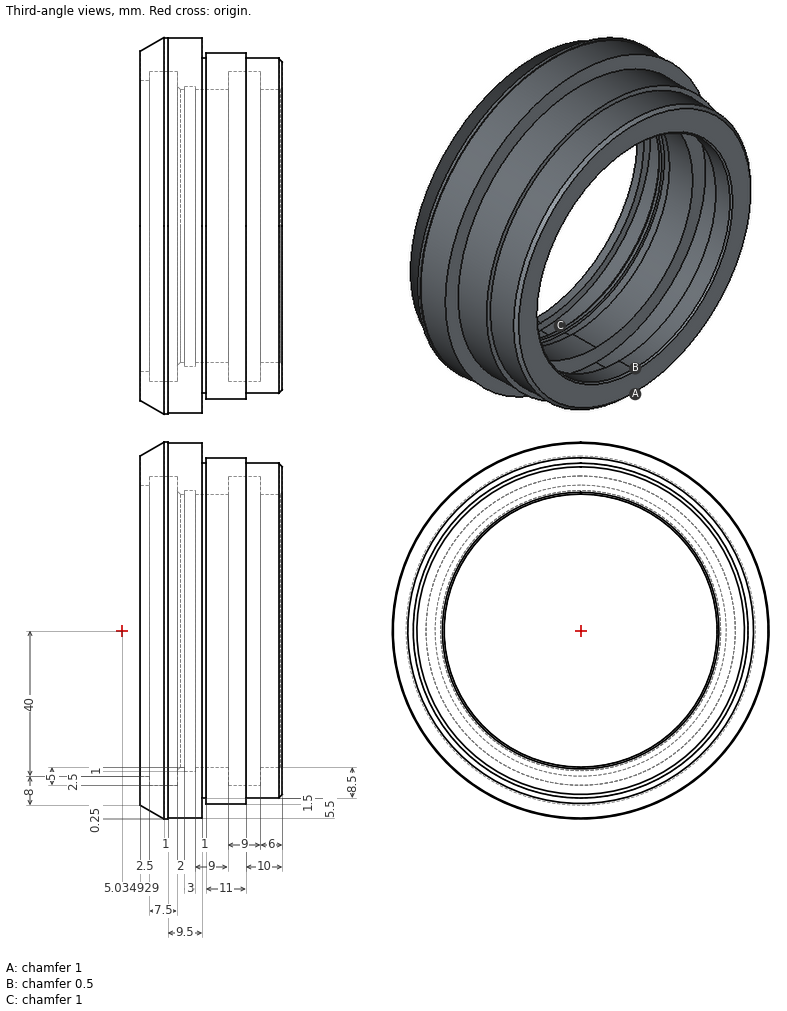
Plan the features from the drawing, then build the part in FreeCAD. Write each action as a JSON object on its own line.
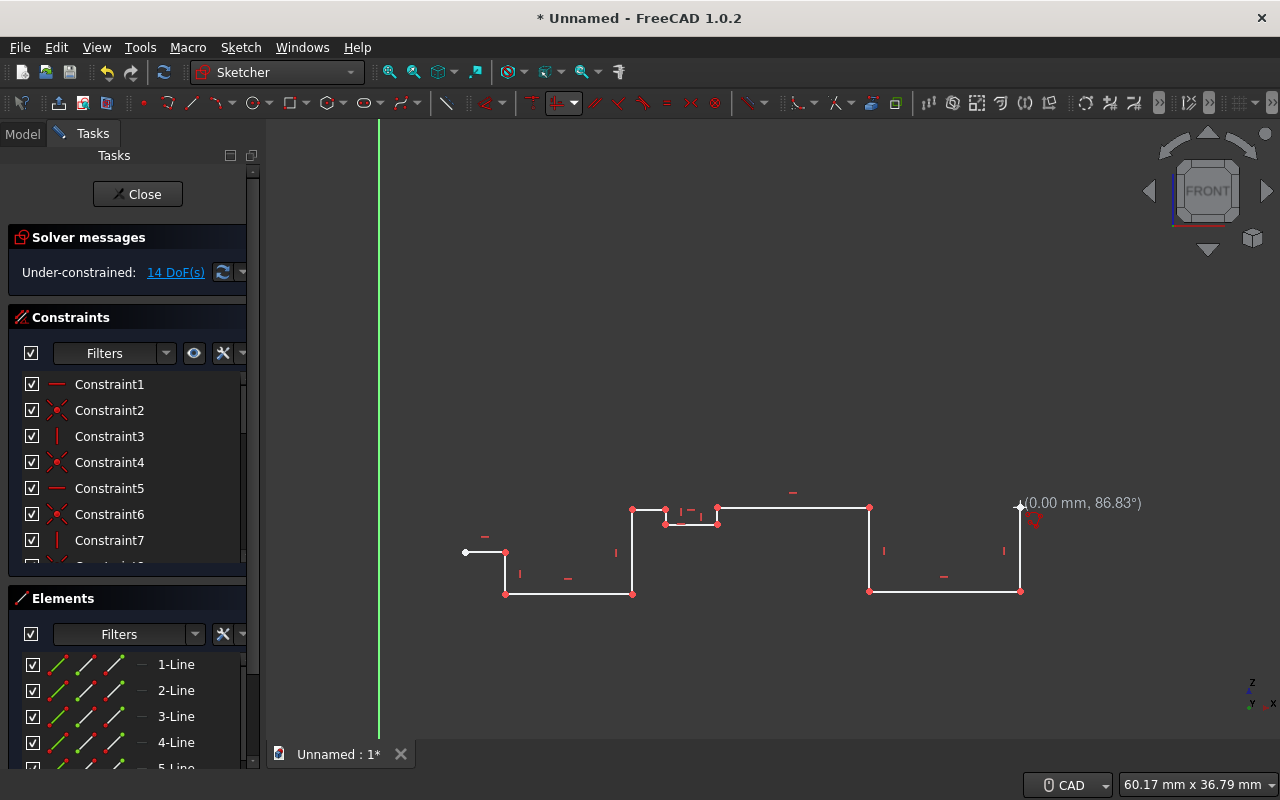
{"action": "scroll", "coordinate": [667, 525], "scroll_direction": "down", "scroll_amount": 4}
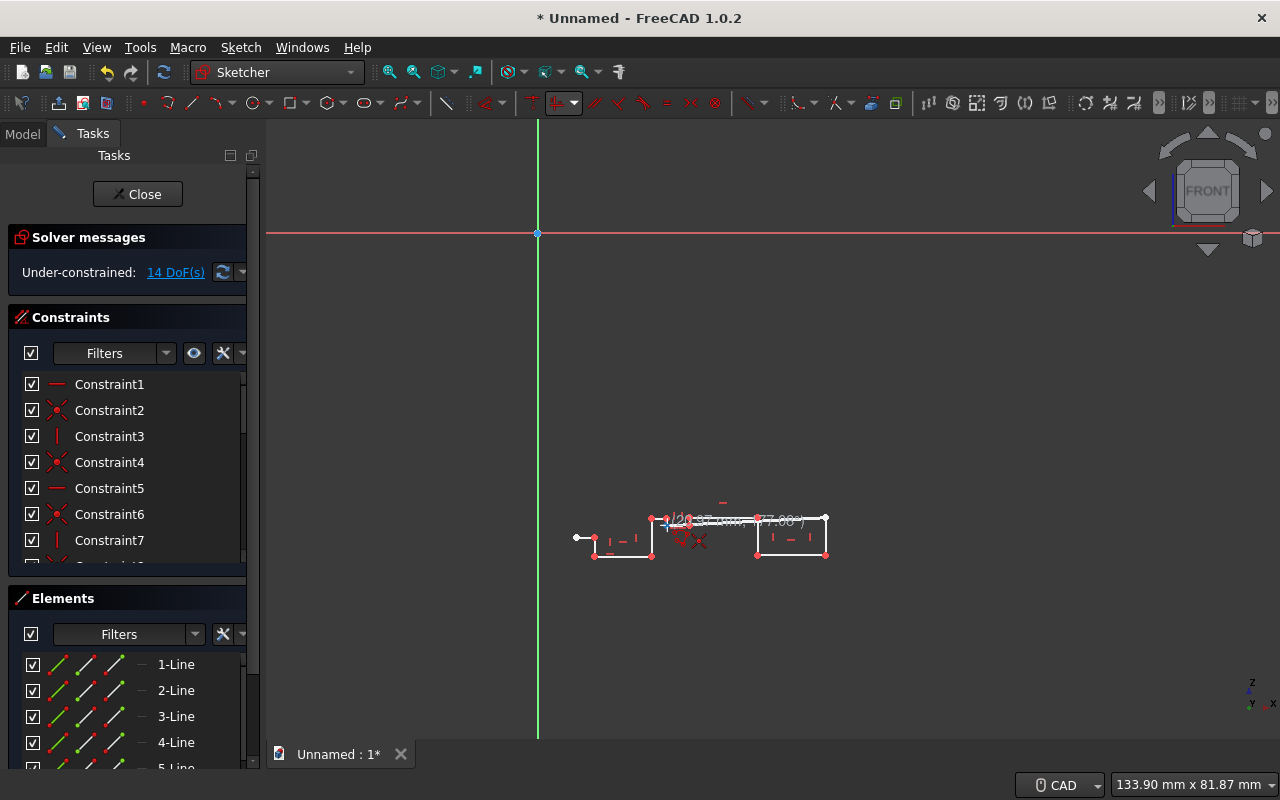
{"action": "left_click", "coordinate": [871, 517]}
{"action": "left_click", "coordinate": [871, 582]}
{"action": "left_click", "coordinate": [796, 582]}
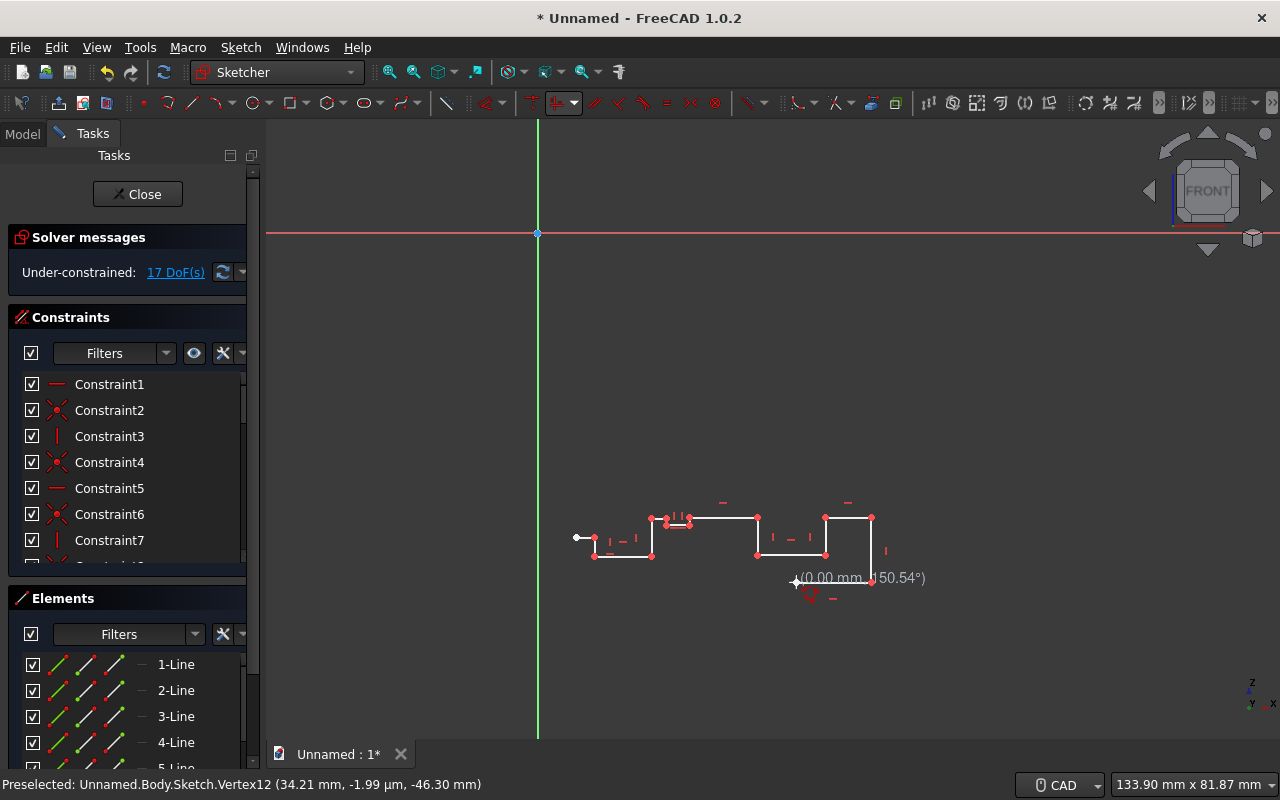
{"action": "scroll", "coordinate": [796, 593], "scroll_direction": "up", "scroll_amount": 2}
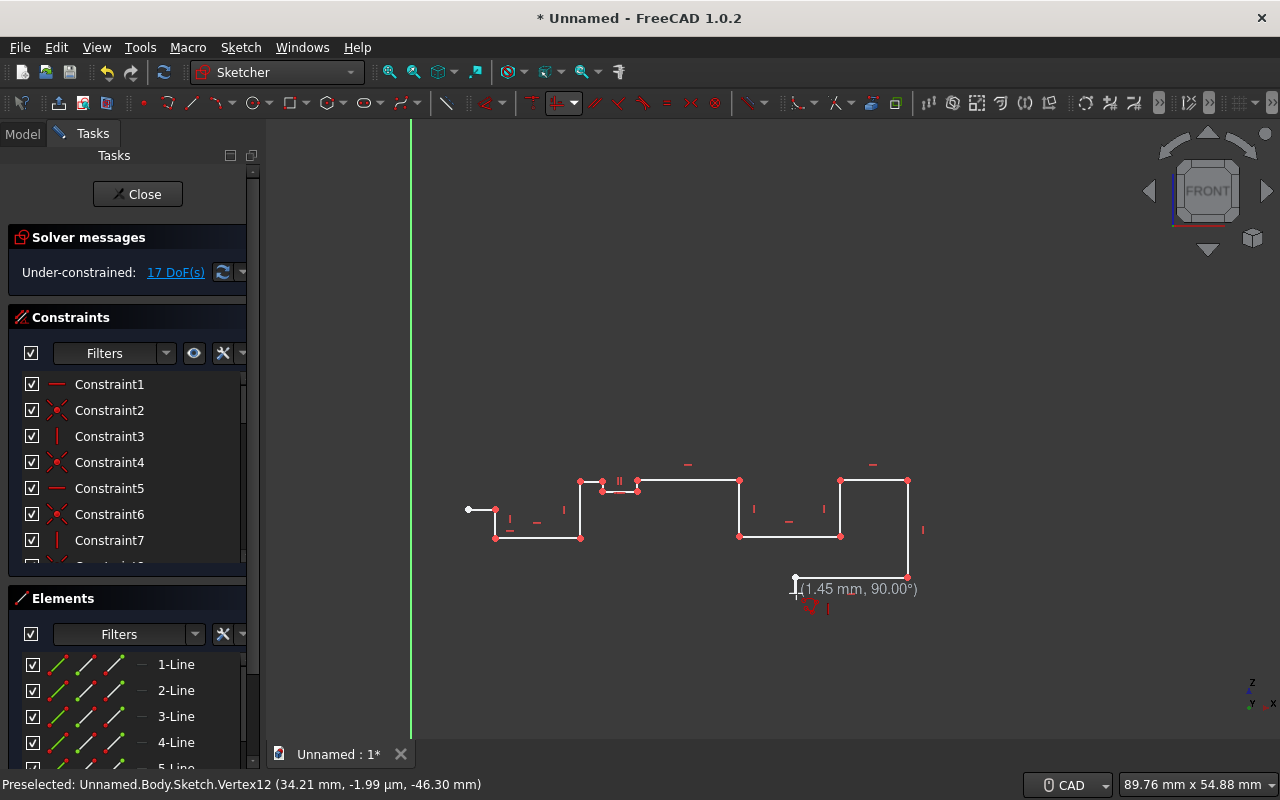
{"action": "left_click", "coordinate": [796, 593]}
{"action": "left_click", "coordinate": [671, 593]}
{"action": "left_click", "coordinate": [671, 576]}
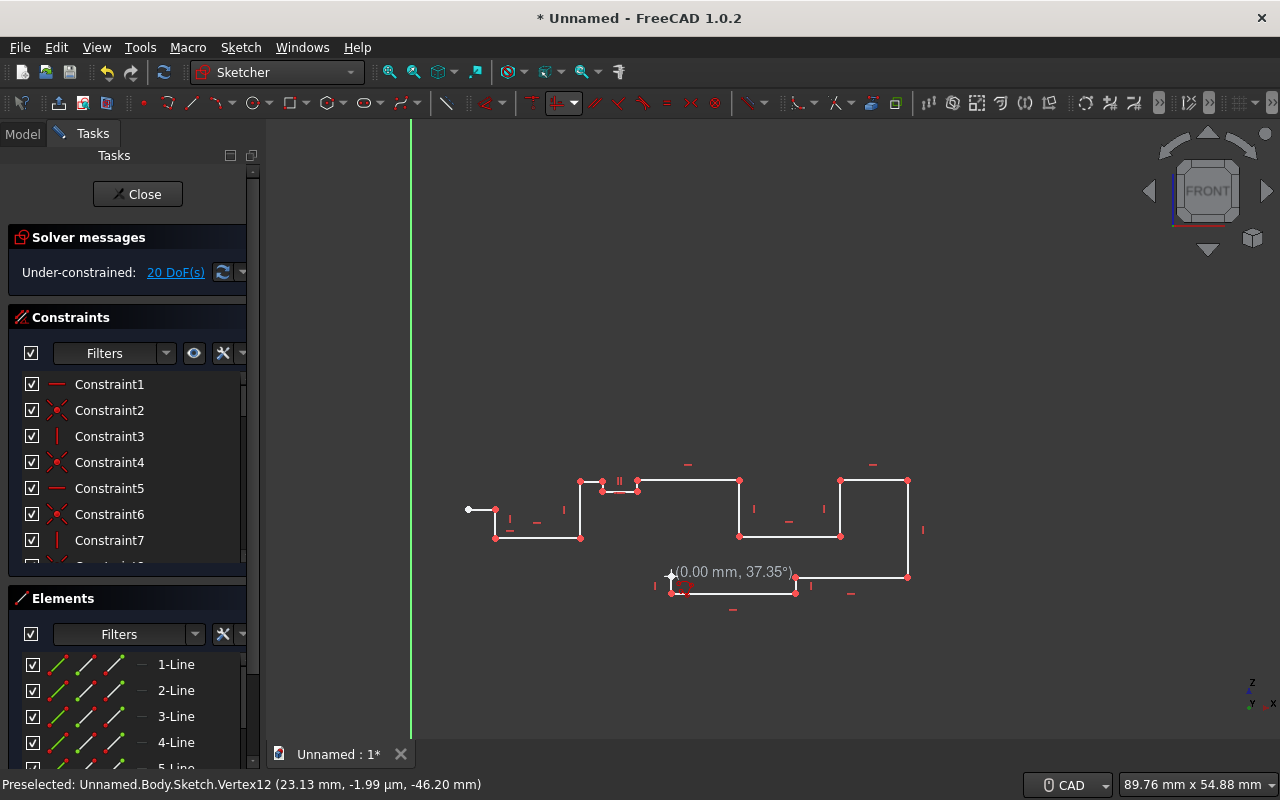
{"action": "scroll", "coordinate": [660, 576], "scroll_direction": "up", "scroll_amount": 2}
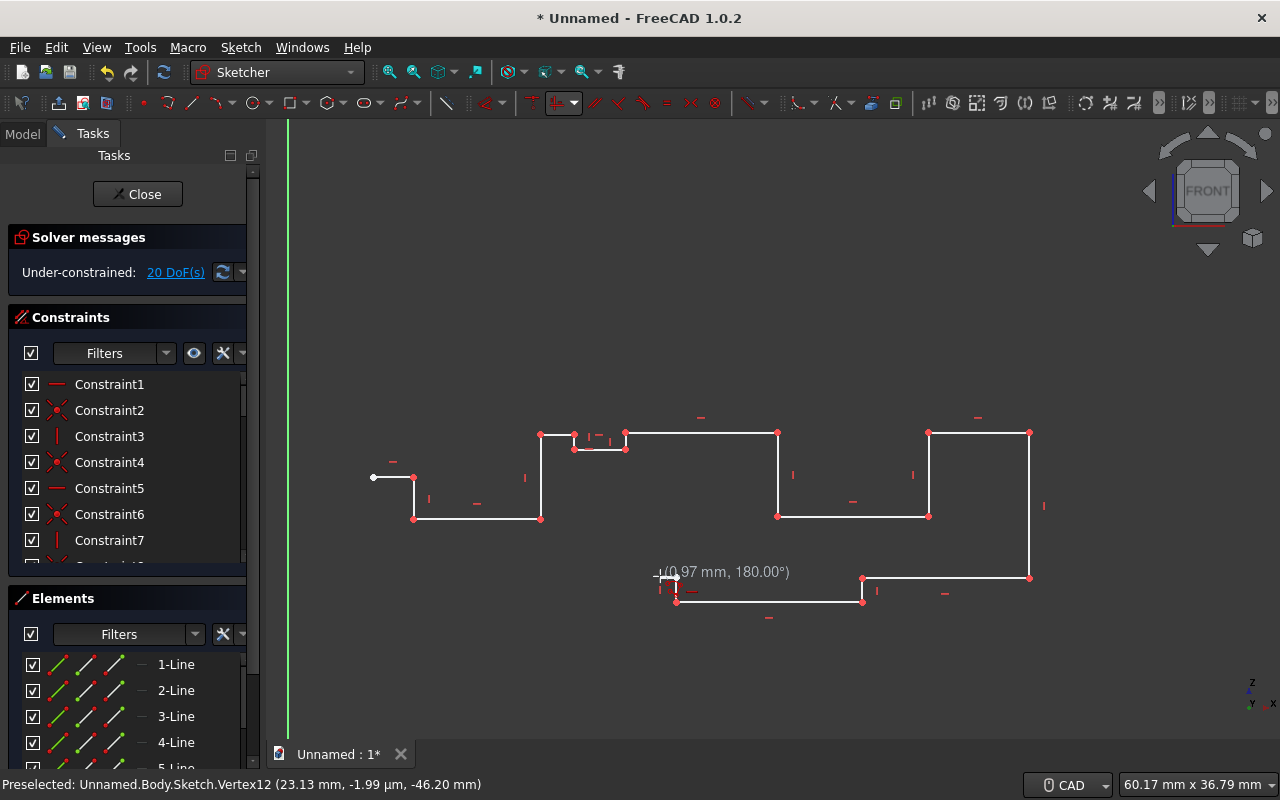
{"action": "left_click", "coordinate": [659, 576]}
{"action": "left_click", "coordinate": [659, 668]}
{"action": "left_click", "coordinate": [499, 668]}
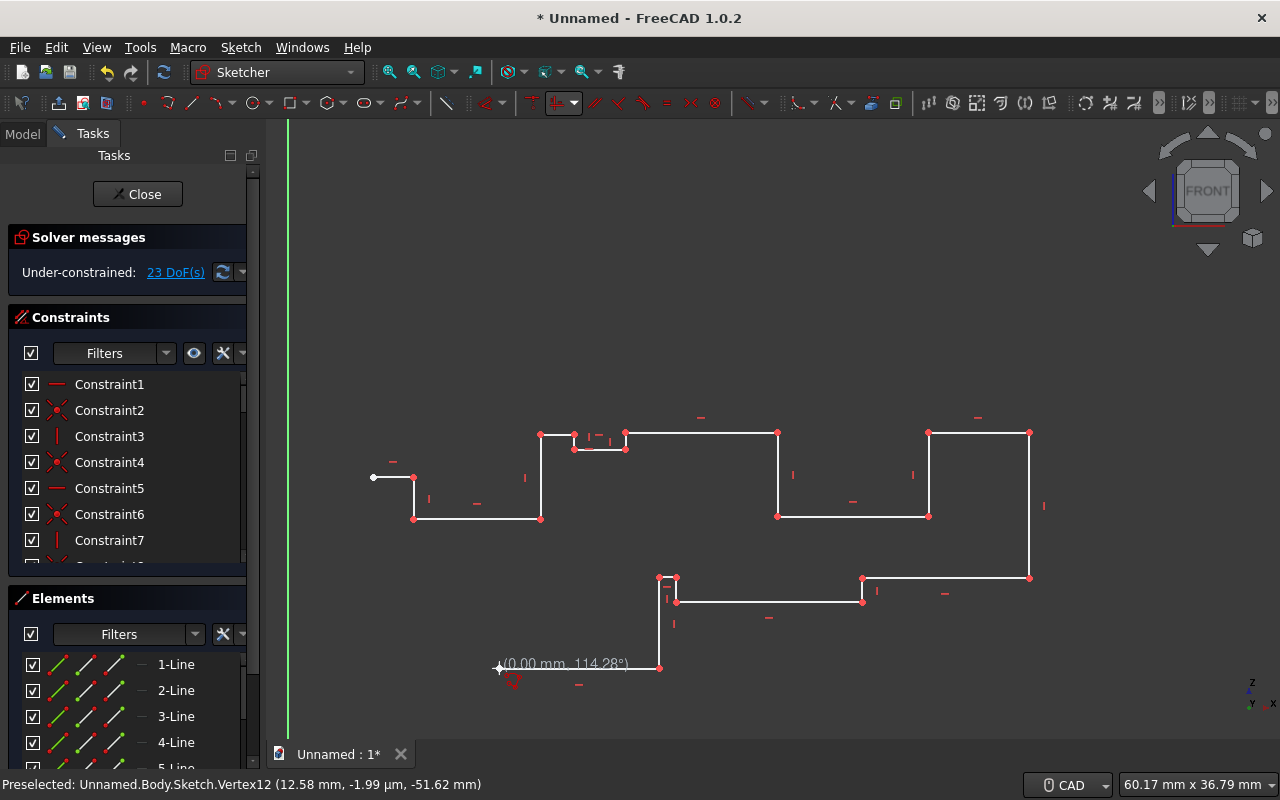
{"action": "scroll", "coordinate": [499, 672], "scroll_direction": "up", "scroll_amount": 7}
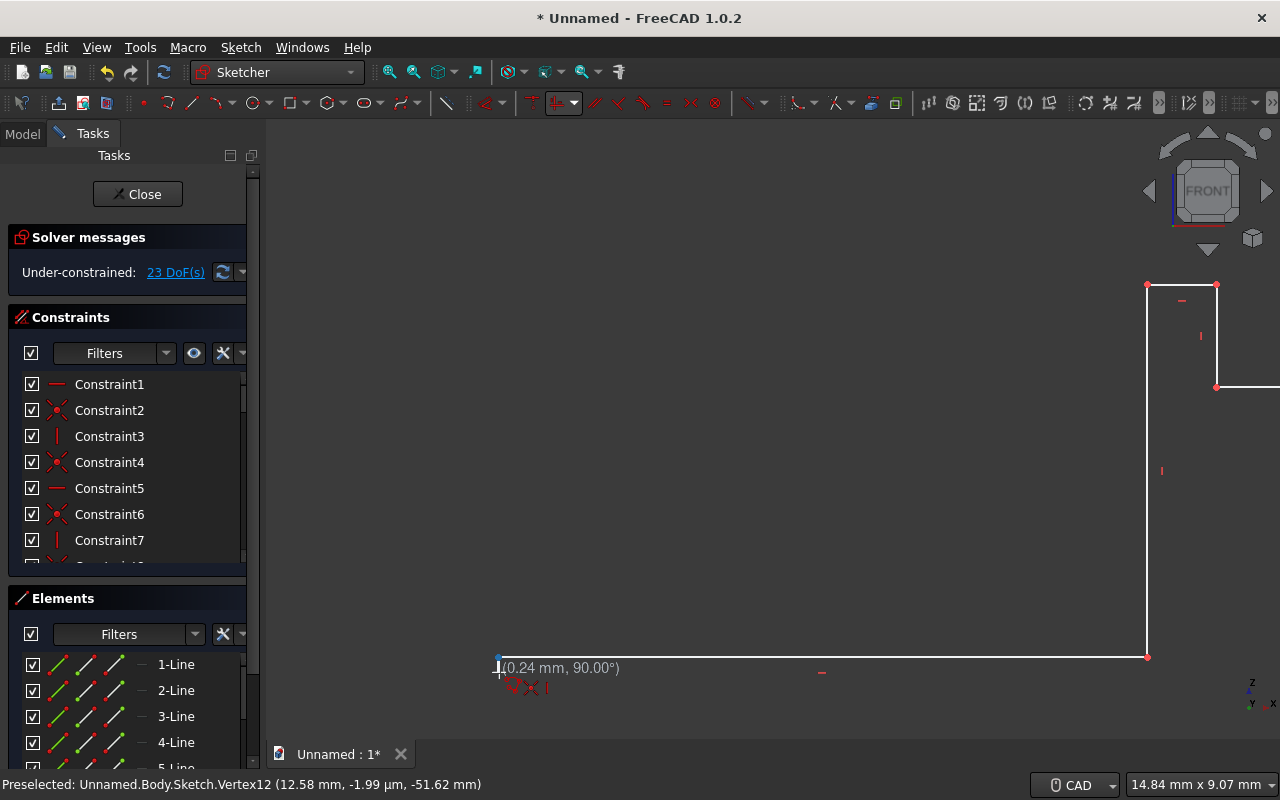
{"action": "left_click", "coordinate": [498, 670]}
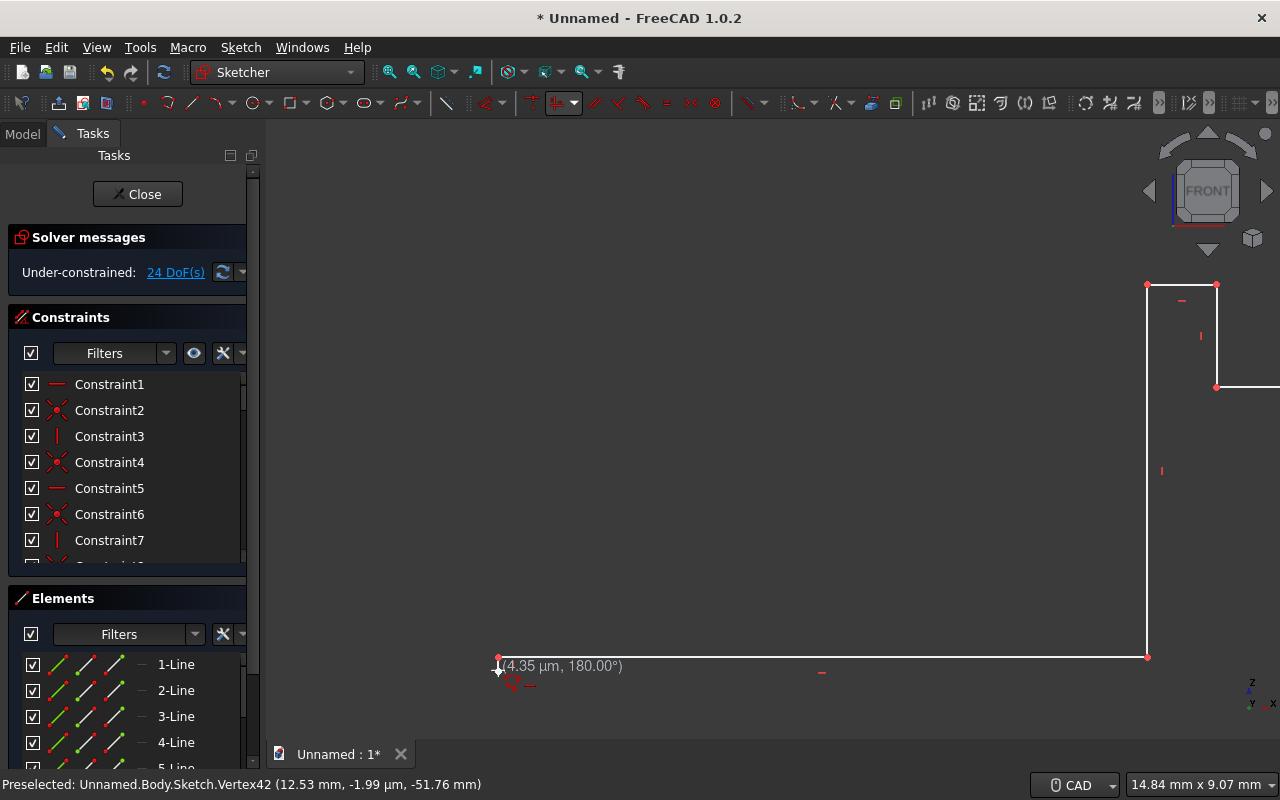
{"action": "scroll", "coordinate": [649, 619], "scroll_direction": "down", "scroll_amount": 11}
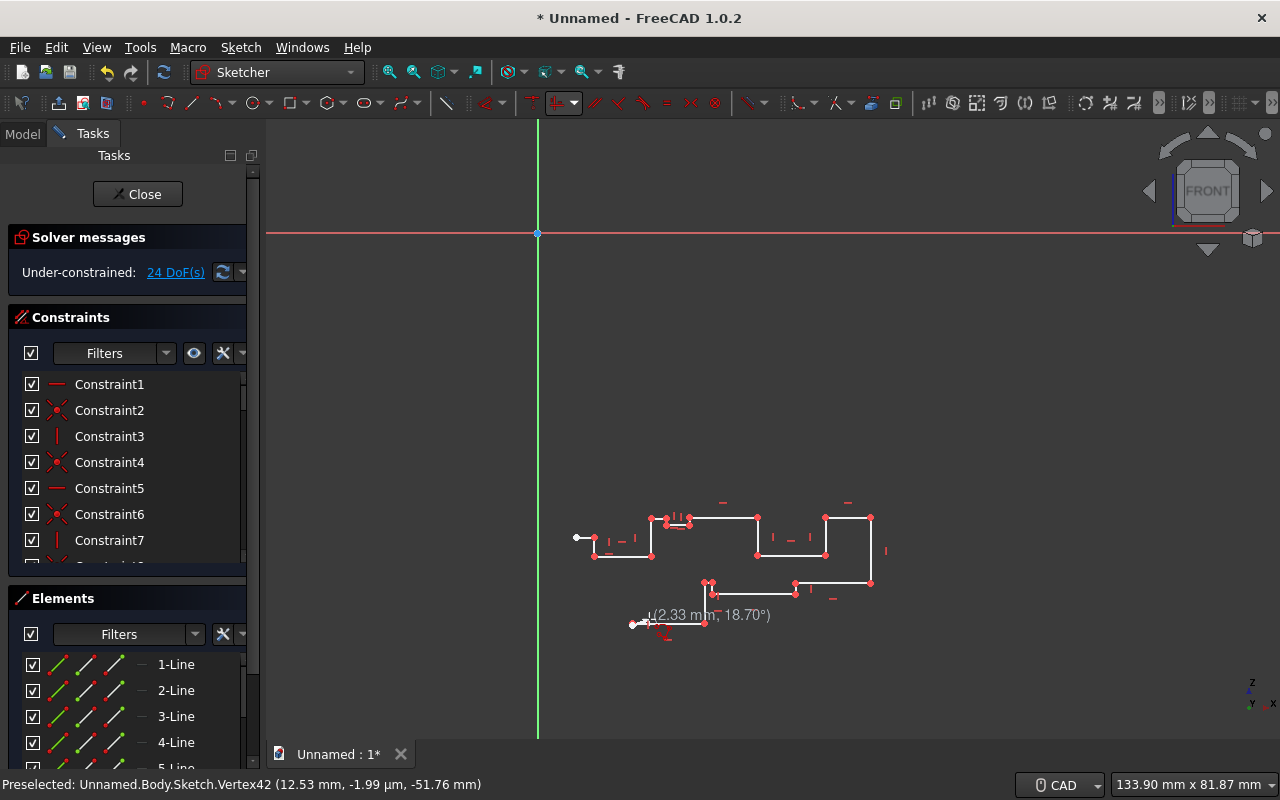
{"action": "scroll", "coordinate": [625, 625], "scroll_direction": "up", "scroll_amount": 4}